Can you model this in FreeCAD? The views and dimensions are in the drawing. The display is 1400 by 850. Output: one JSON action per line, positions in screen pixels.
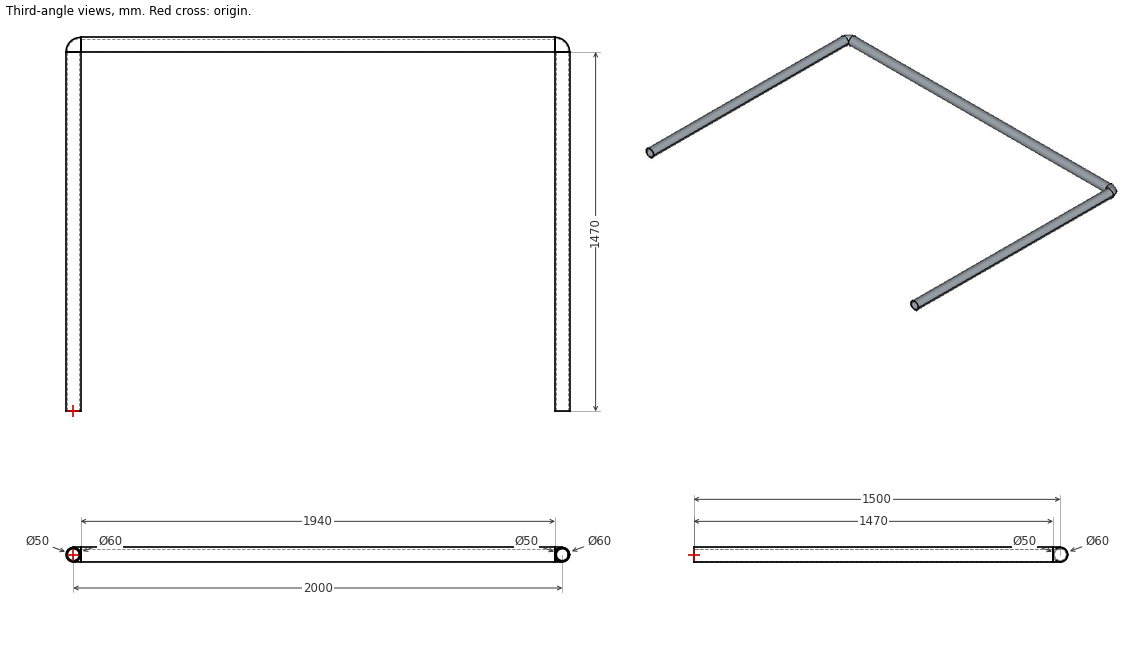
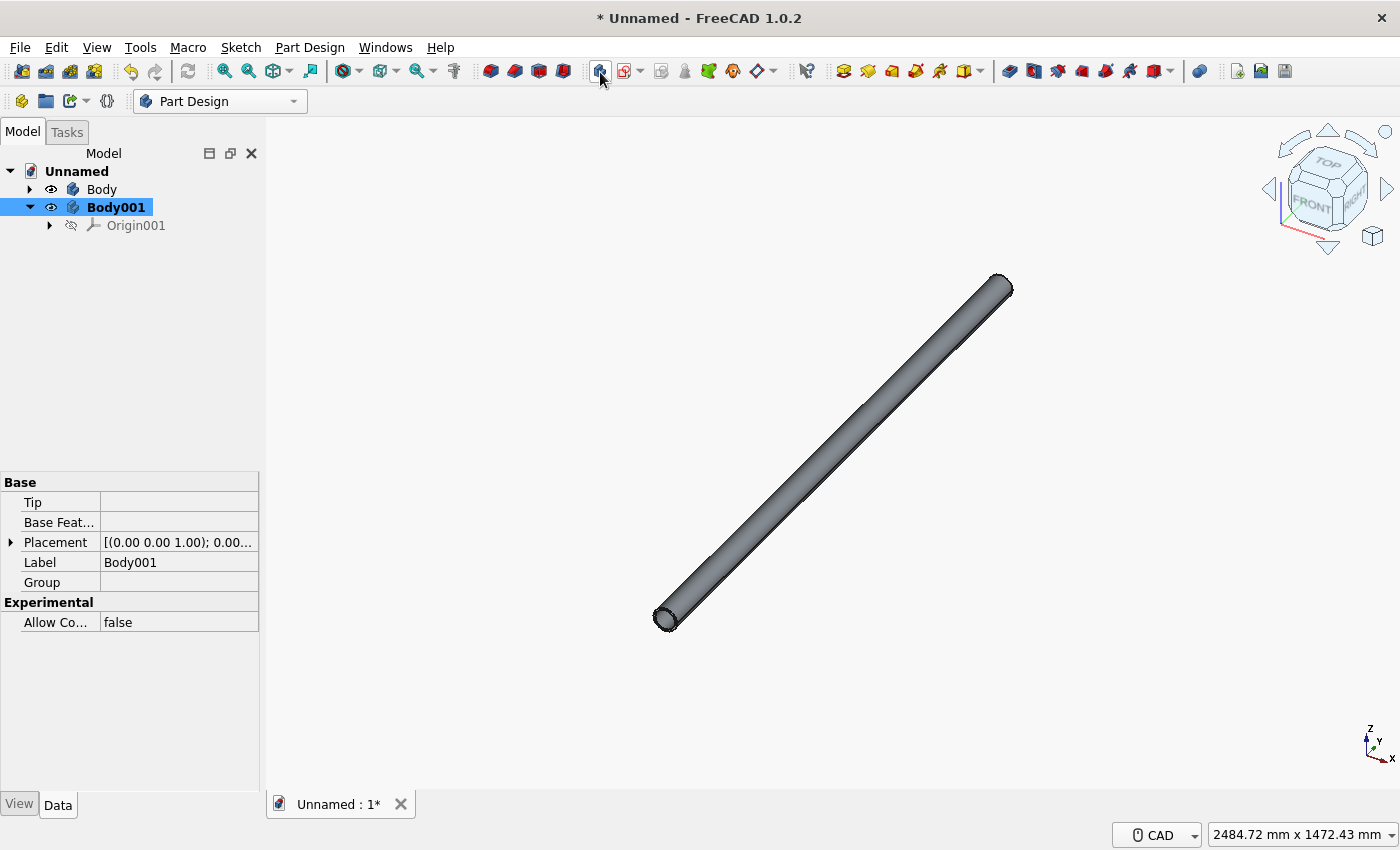
{"action": "left_click", "coordinate": [50, 225]}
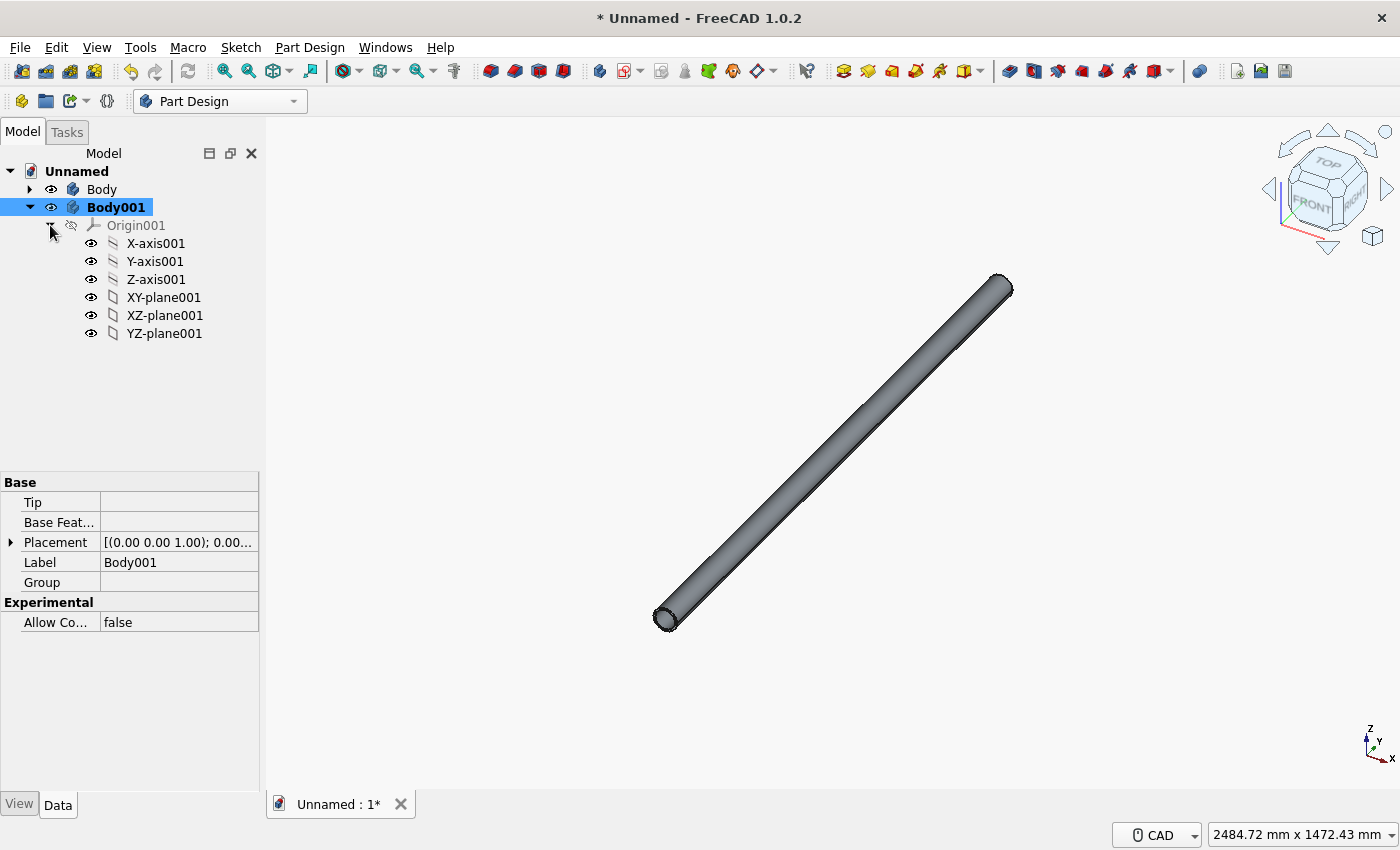
{"action": "left_click", "coordinate": [136, 315]}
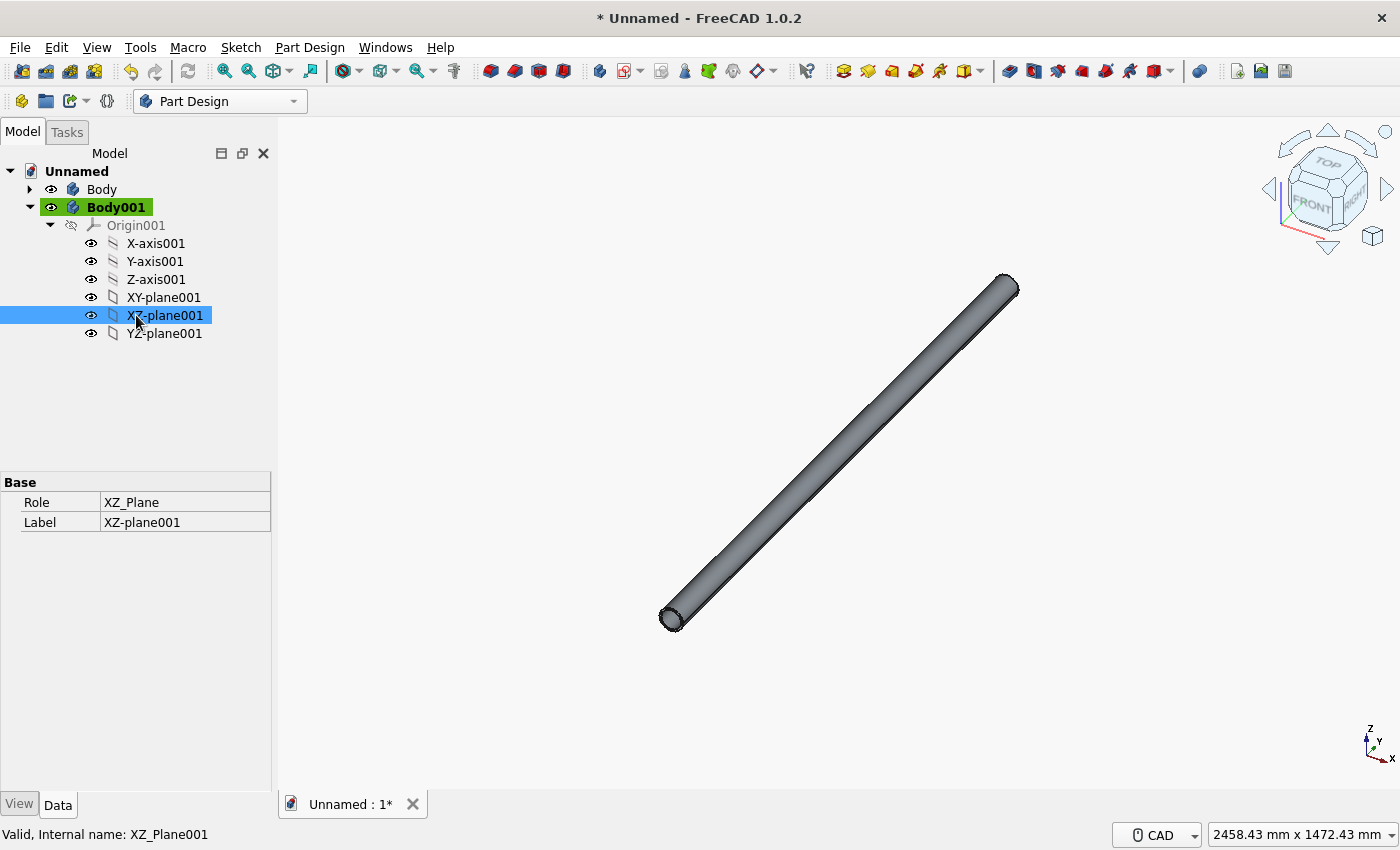
{"action": "left_click", "coordinate": [758, 72]}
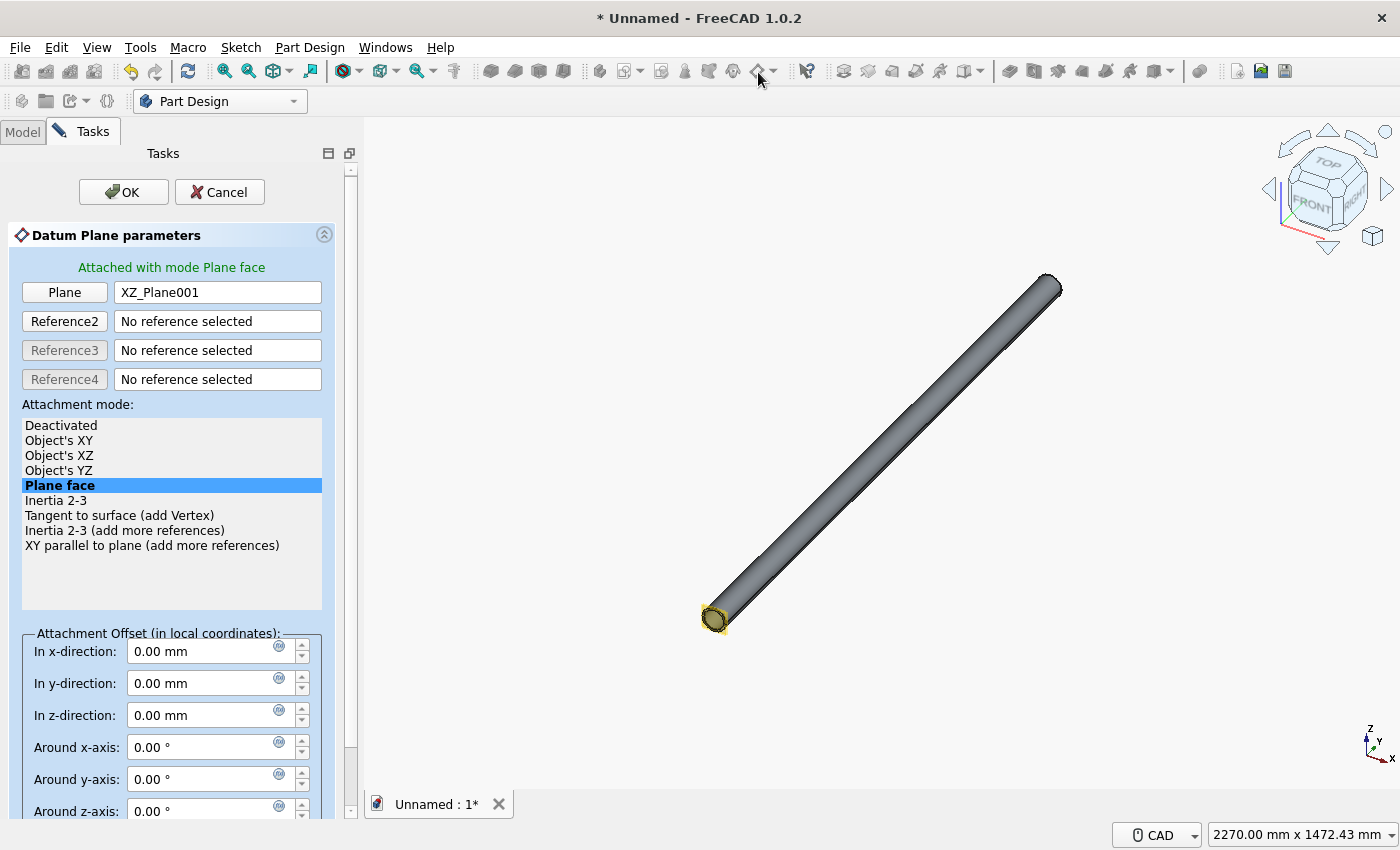
{"action": "triple_click", "coordinate": [210, 715]}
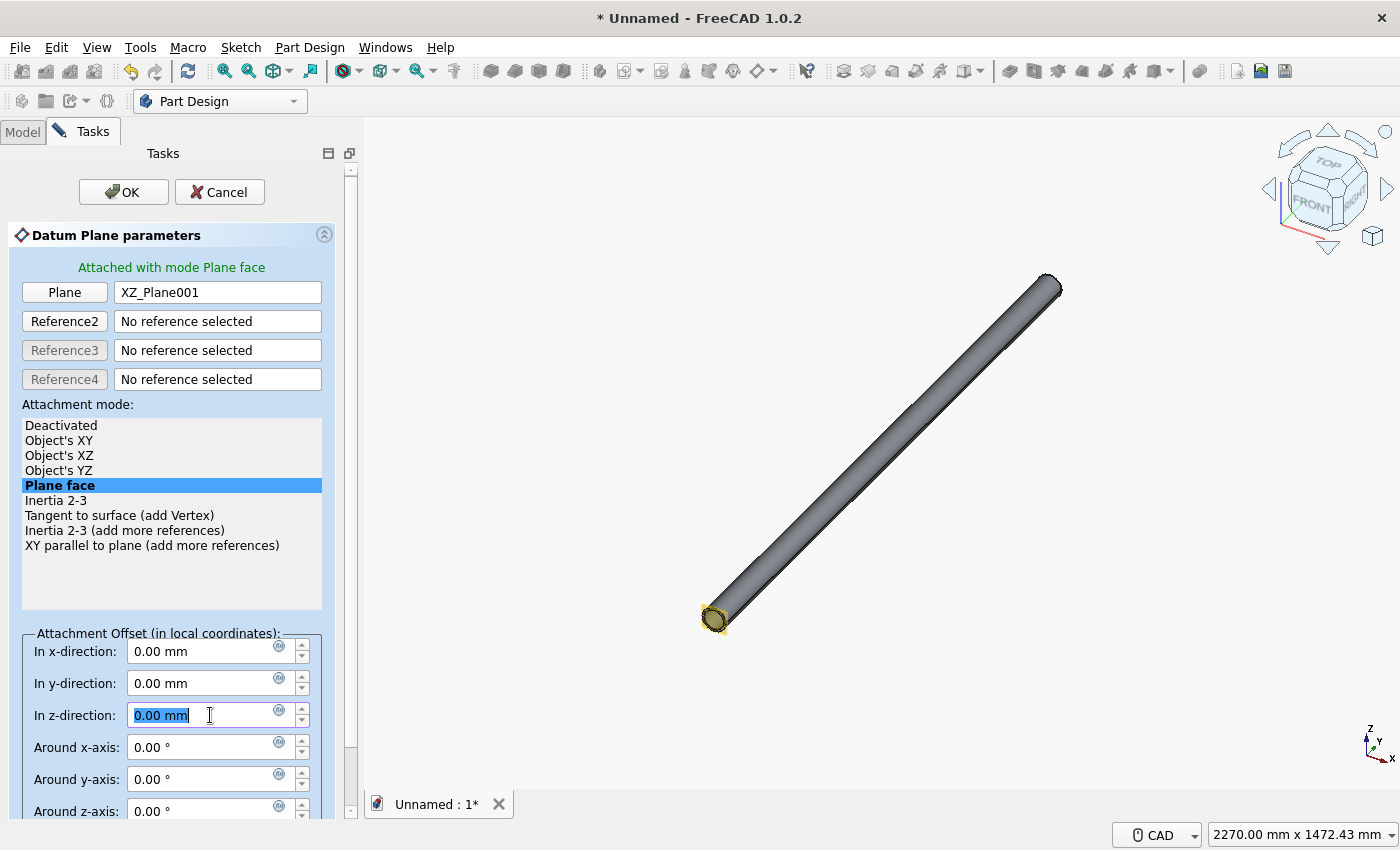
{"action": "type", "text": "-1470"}
{"action": "key", "text": "Tab"}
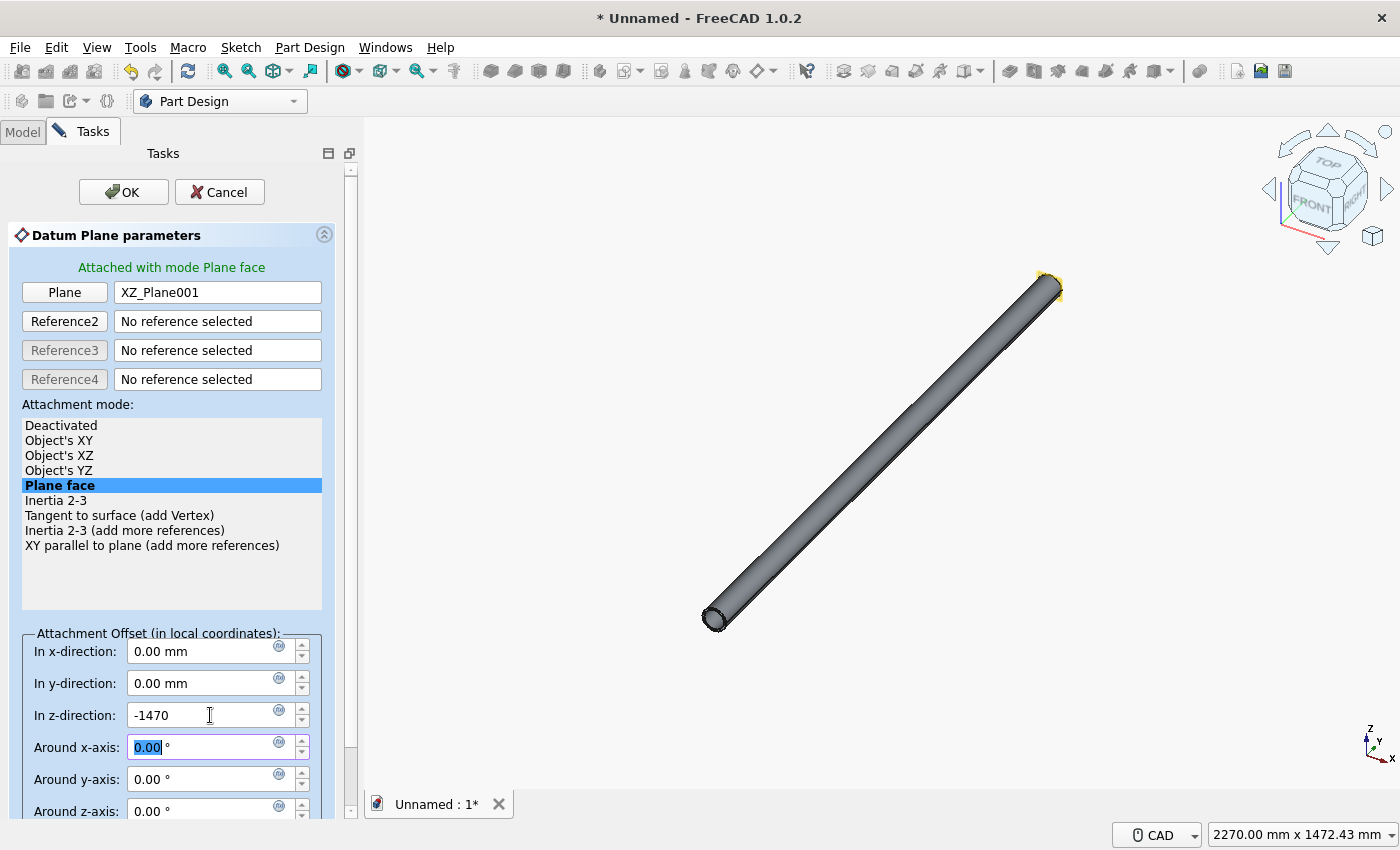
{"action": "left_click", "coordinate": [124, 192]}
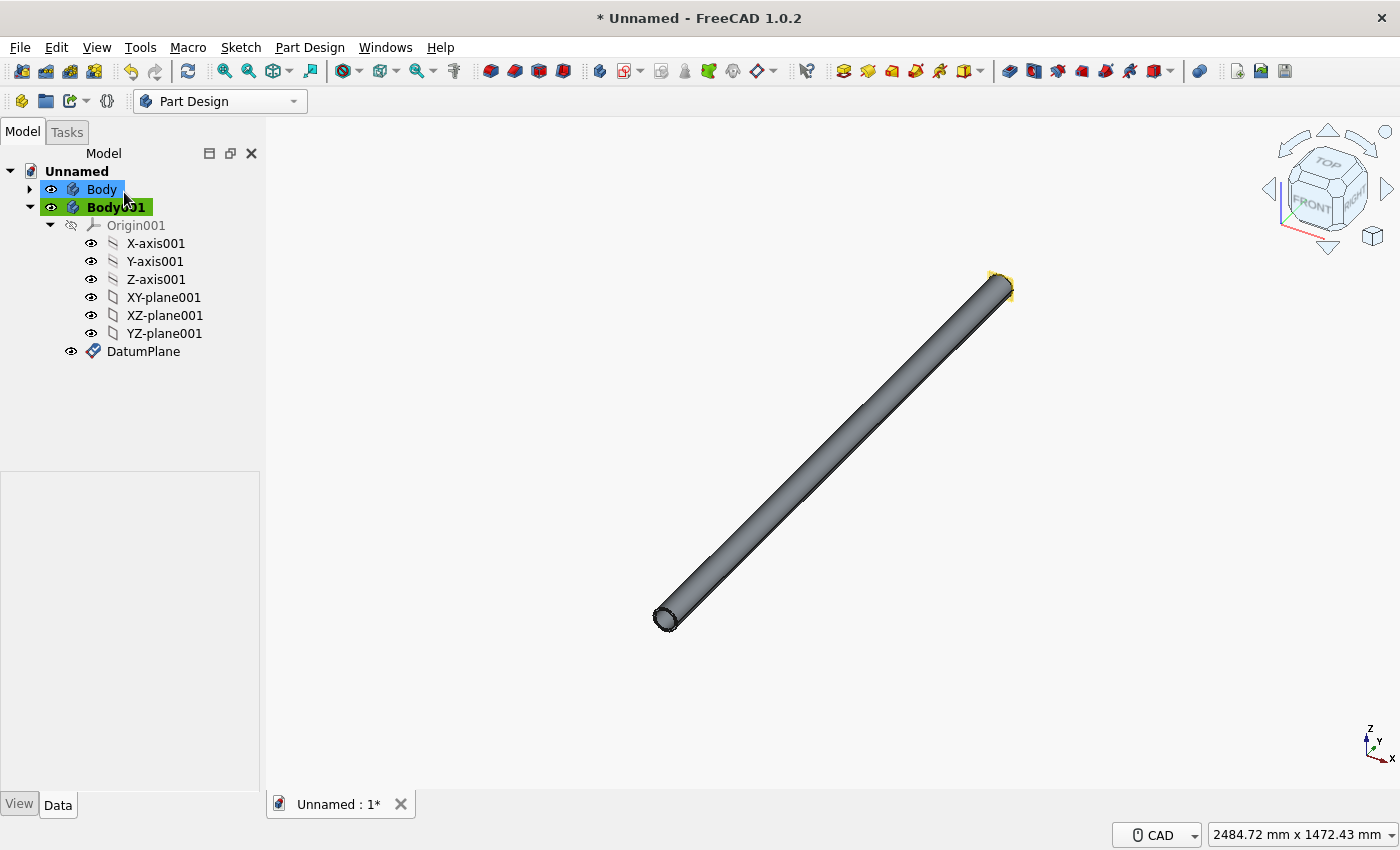
{"action": "left_click", "coordinate": [116, 351]}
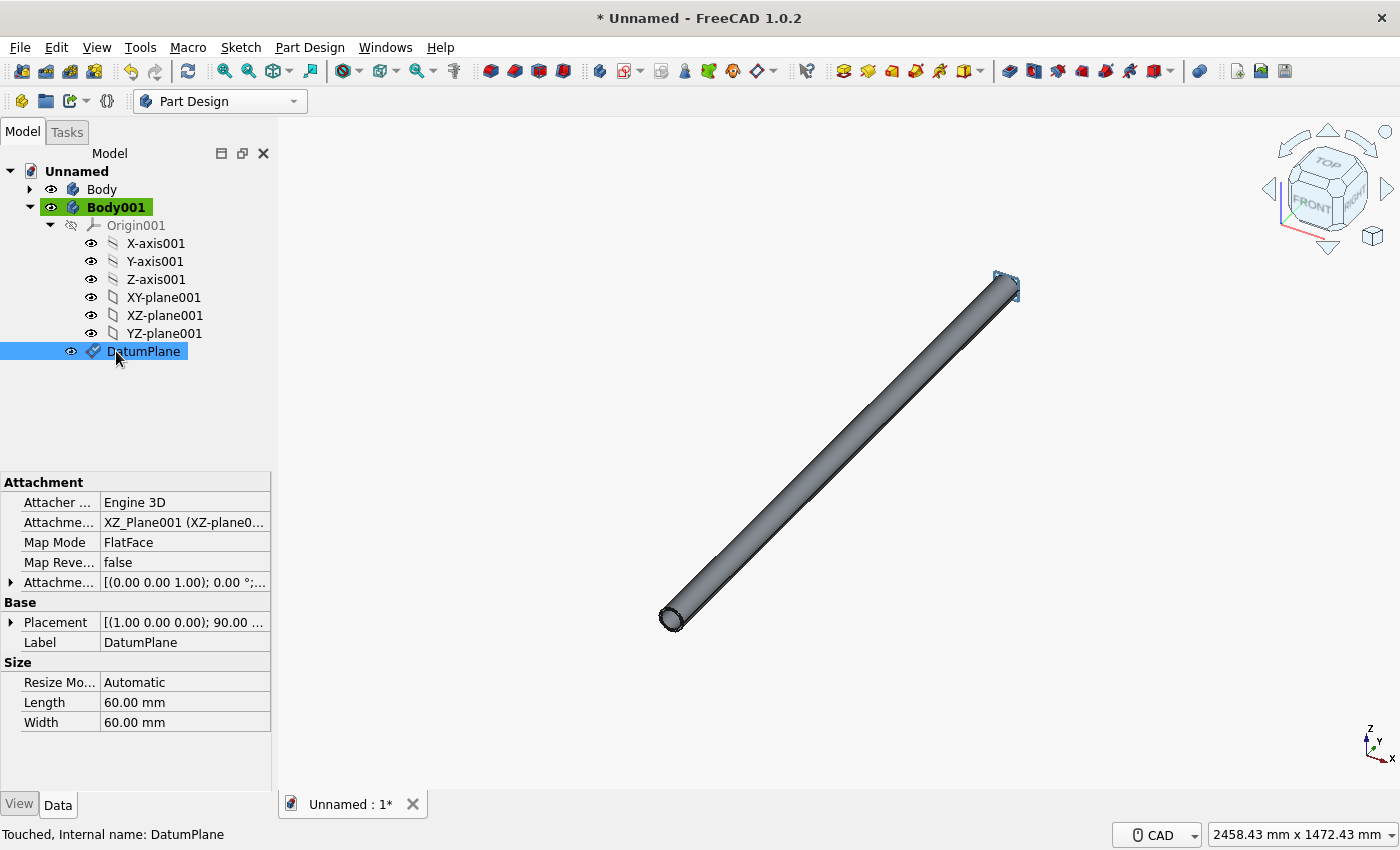
{"action": "left_click", "coordinate": [624, 72]}